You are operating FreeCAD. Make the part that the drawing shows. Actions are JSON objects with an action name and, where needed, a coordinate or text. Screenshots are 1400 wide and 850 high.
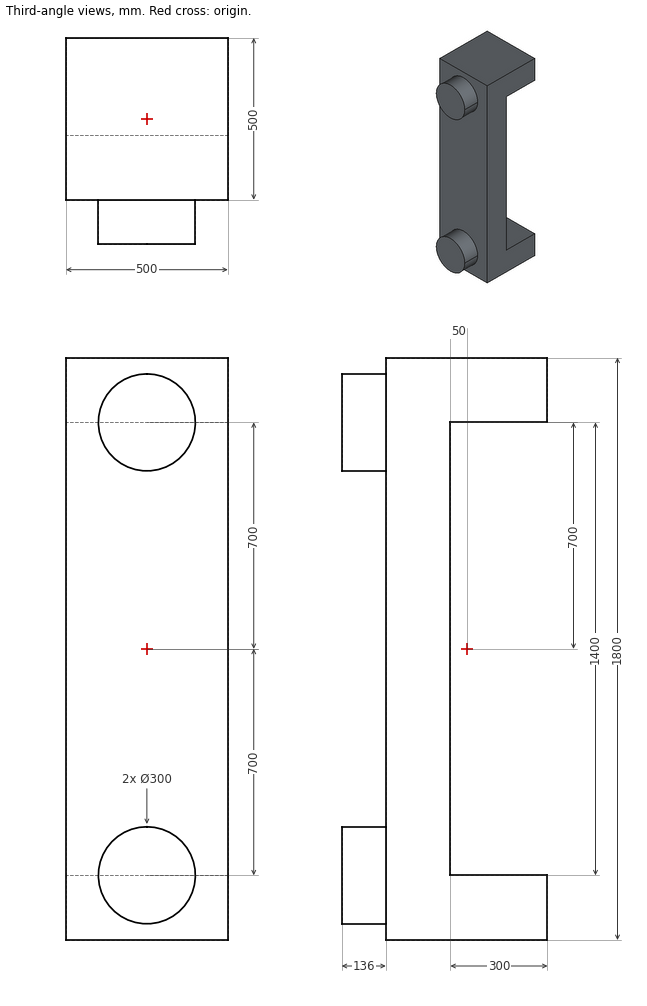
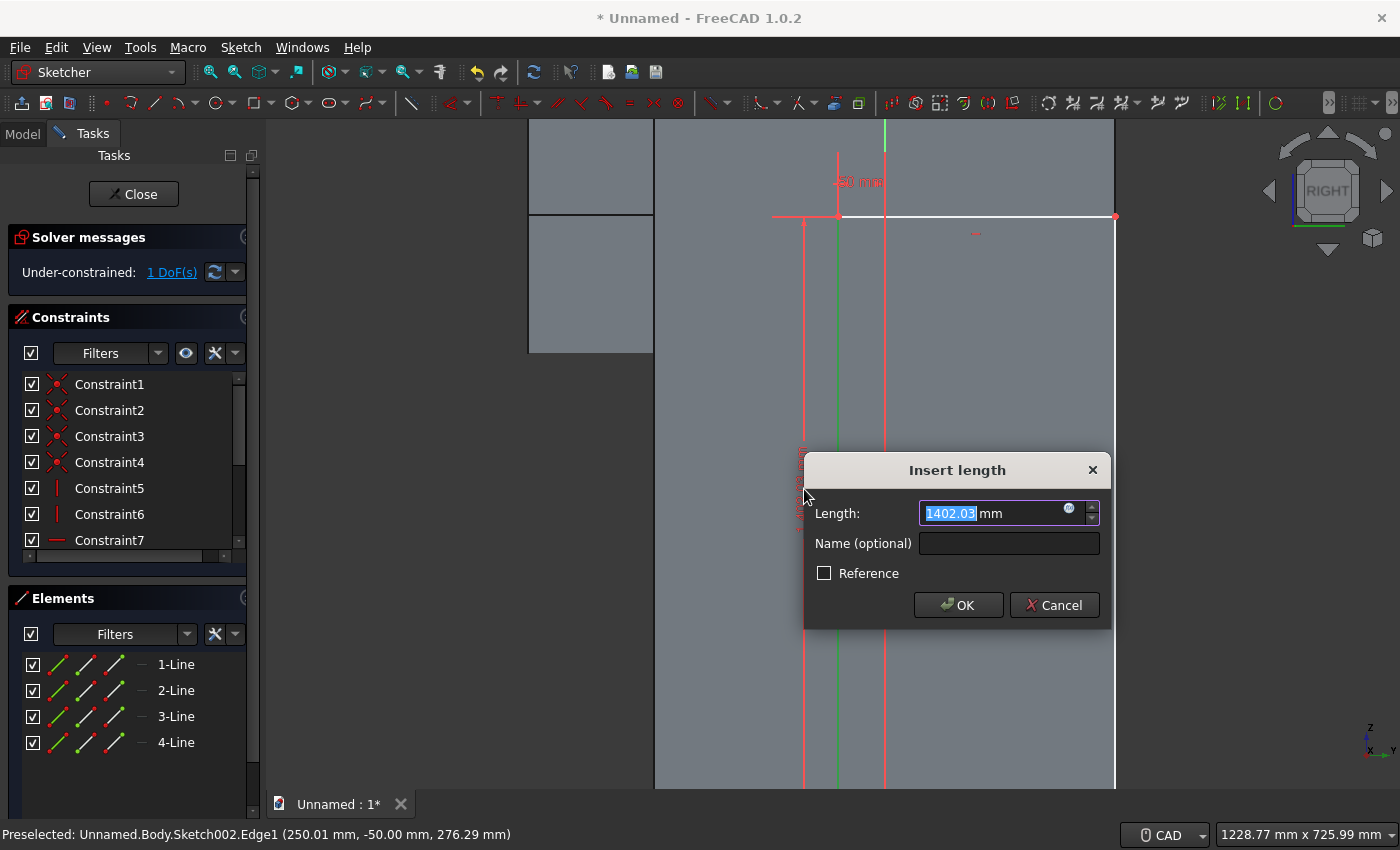
{"action": "type", "text": "1400"}
{"action": "key", "text": "Return"}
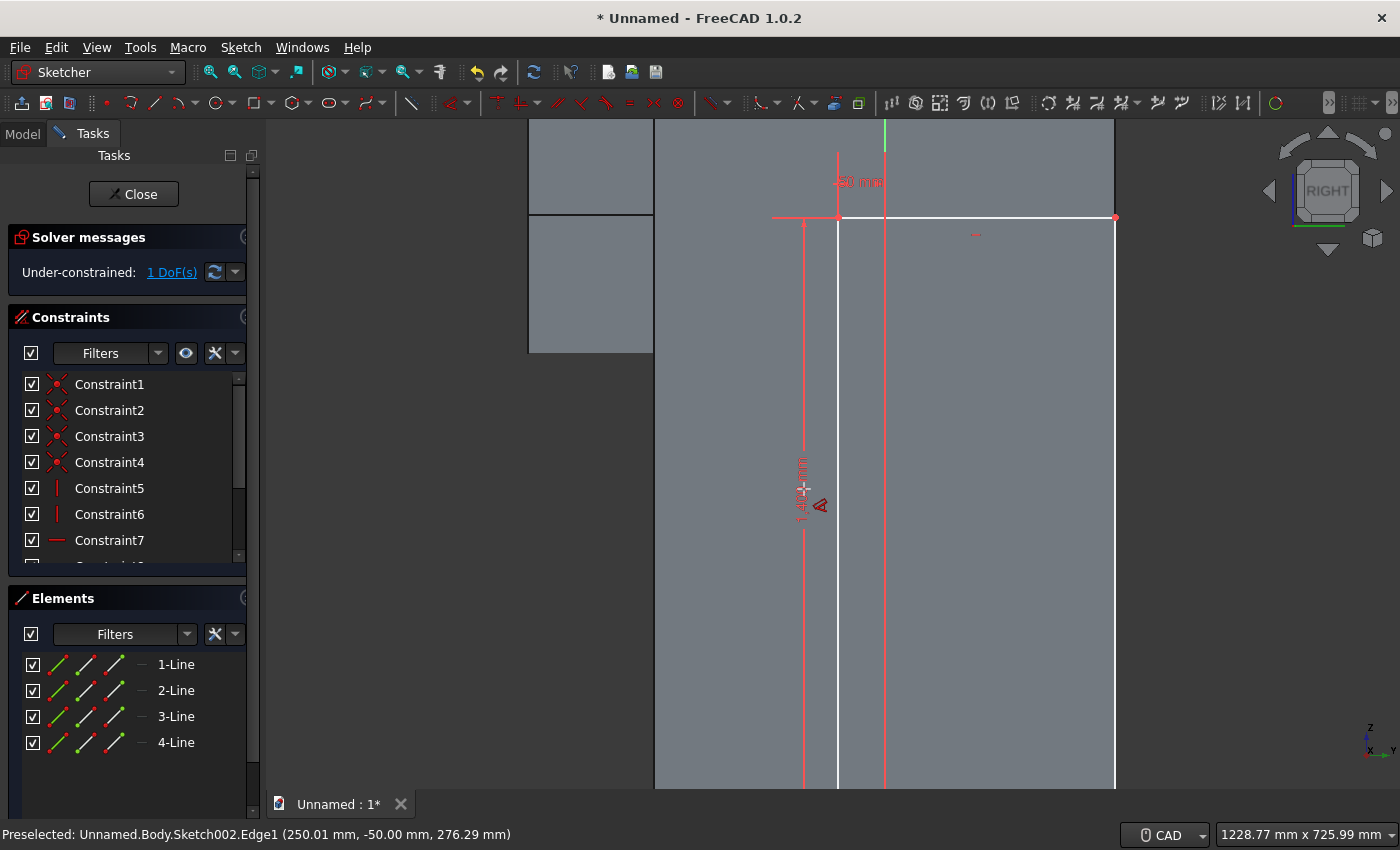
{"action": "left_click", "coordinate": [838, 218]}
{"action": "left_click", "coordinate": [804, 364]}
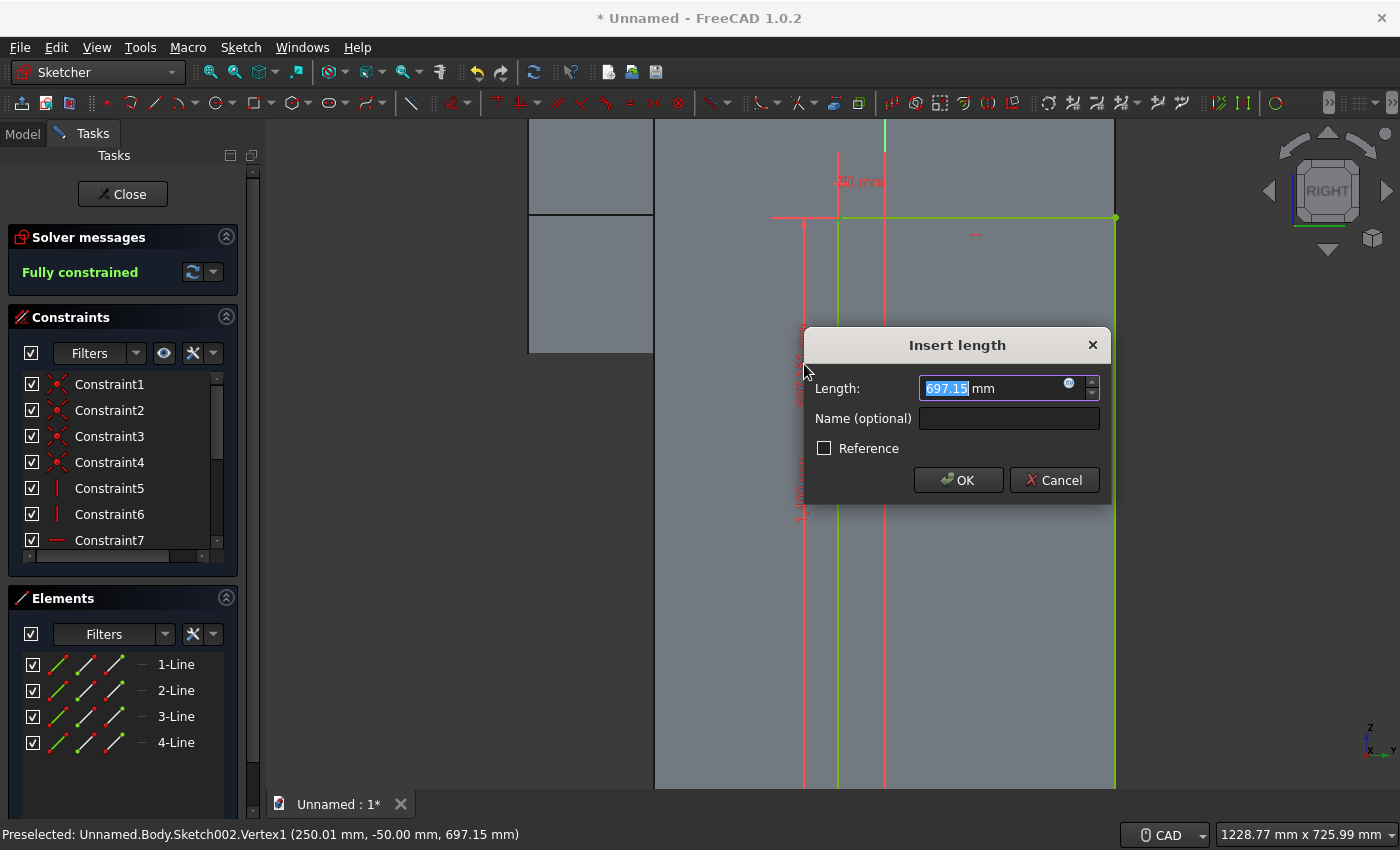
{"action": "type", "text": "700"}
{"action": "key", "text": "Return"}
{"action": "key", "text": "Escape"}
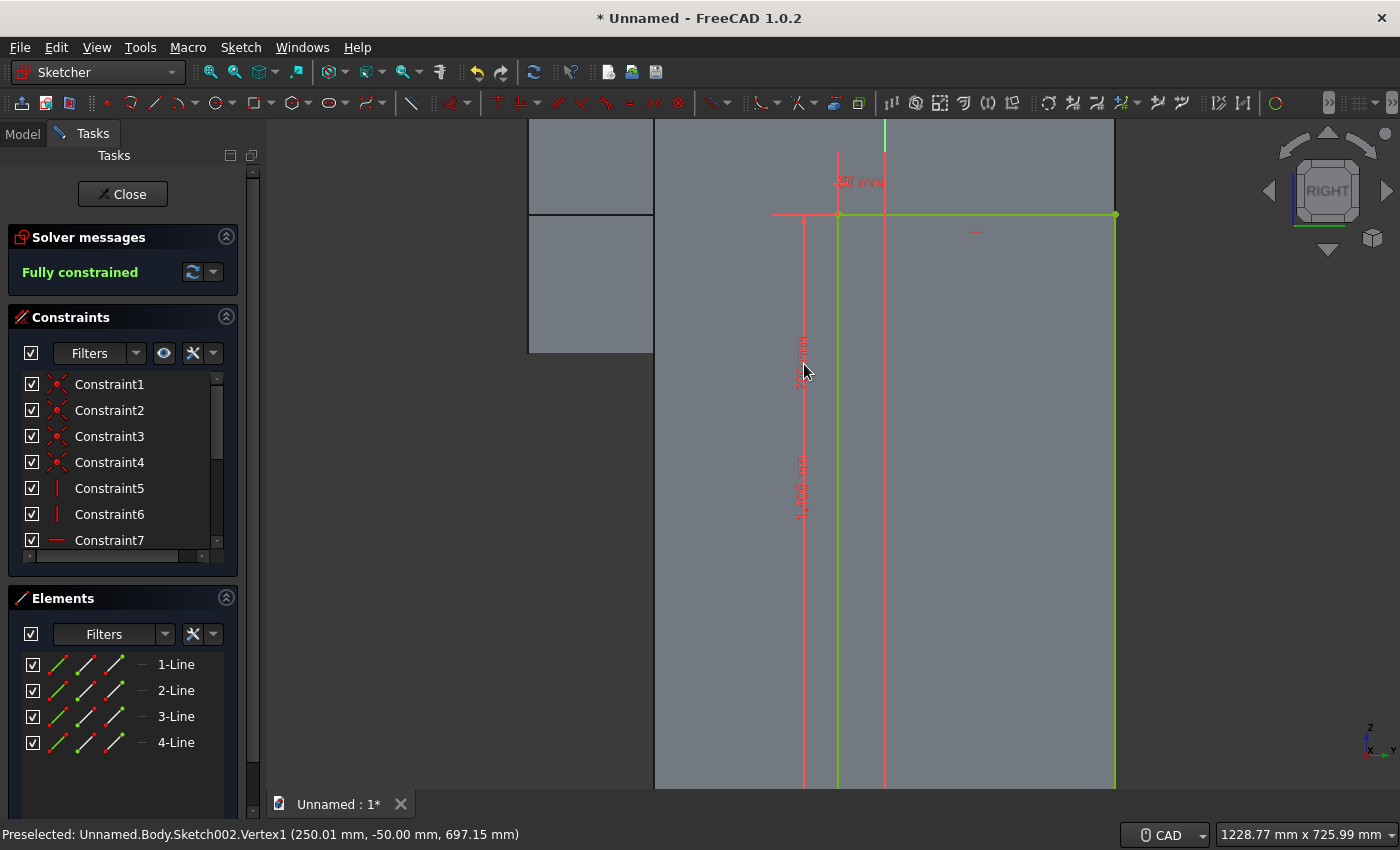
{"action": "left_click", "coordinate": [123, 194]}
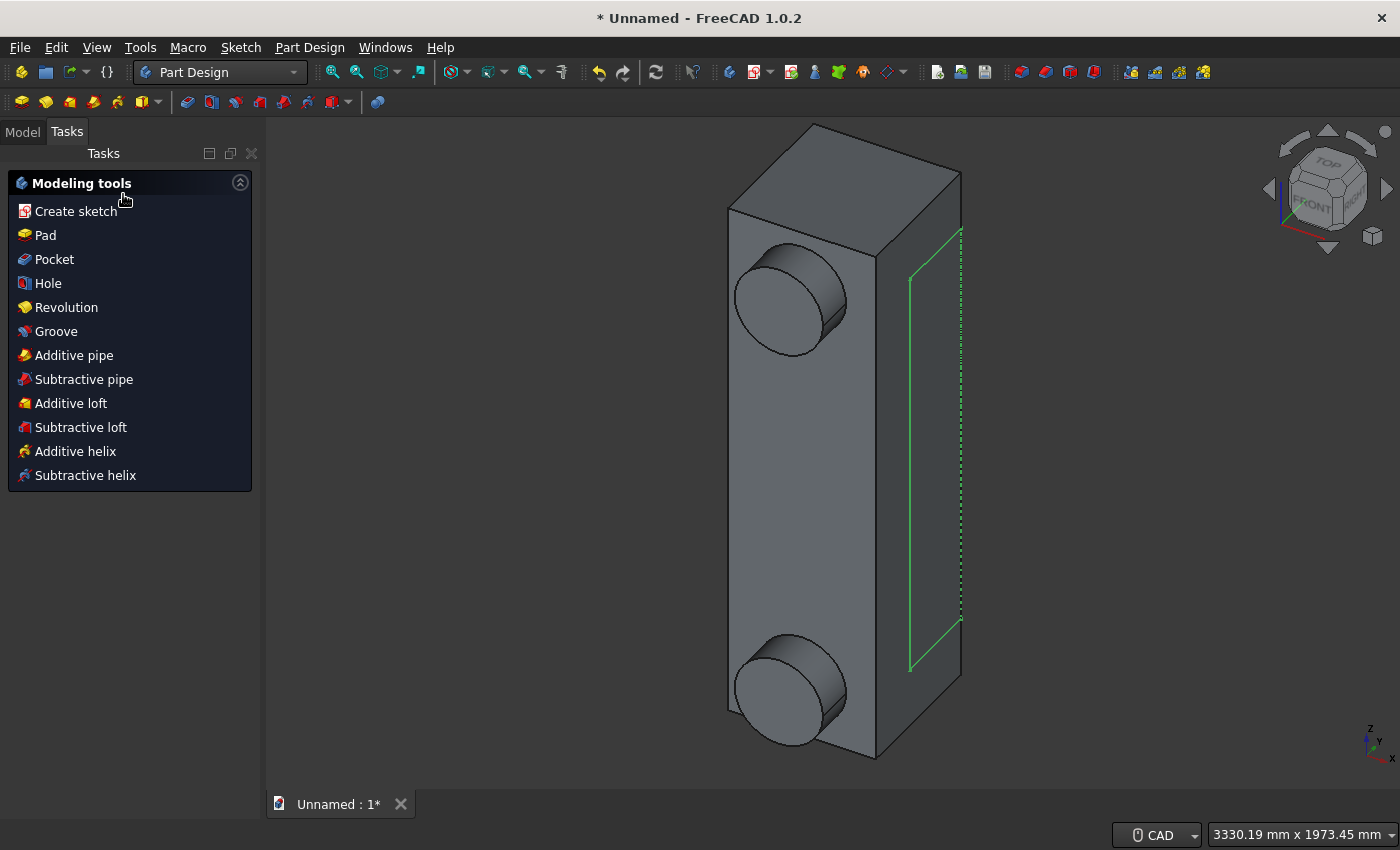
{"action": "left_click", "coordinate": [188, 102]}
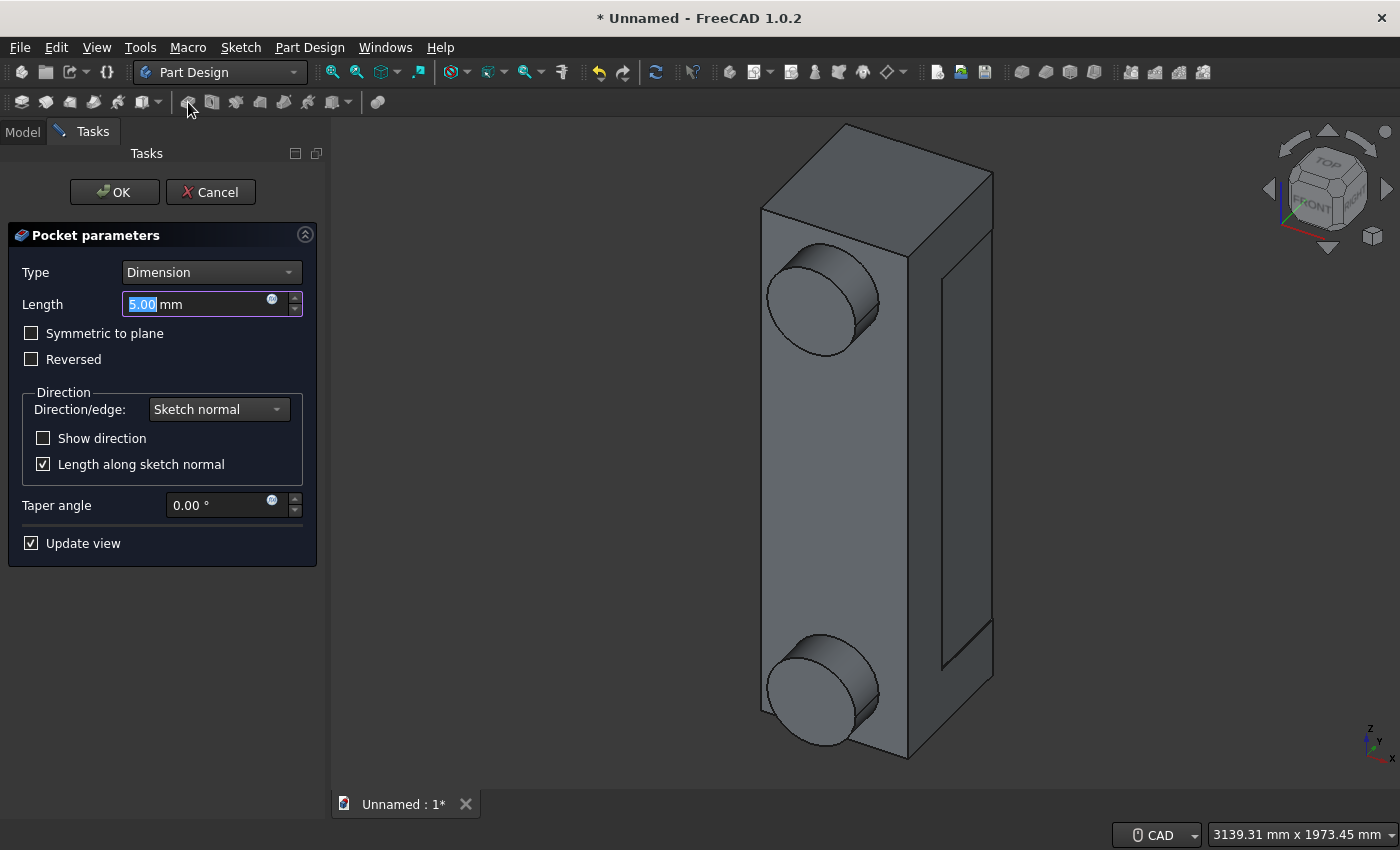
{"action": "left_click", "coordinate": [212, 272]}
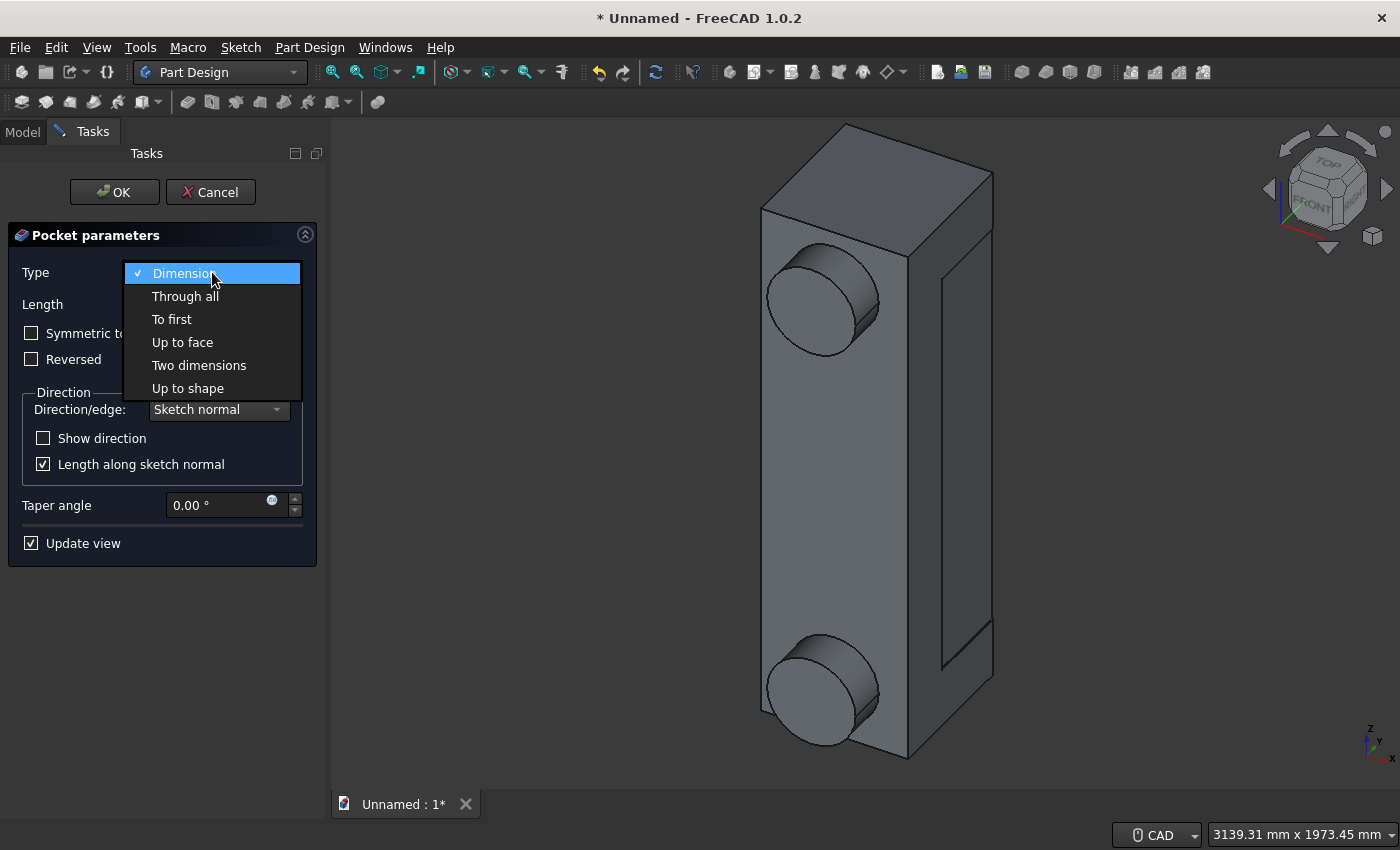
{"action": "left_click", "coordinate": [212, 296]}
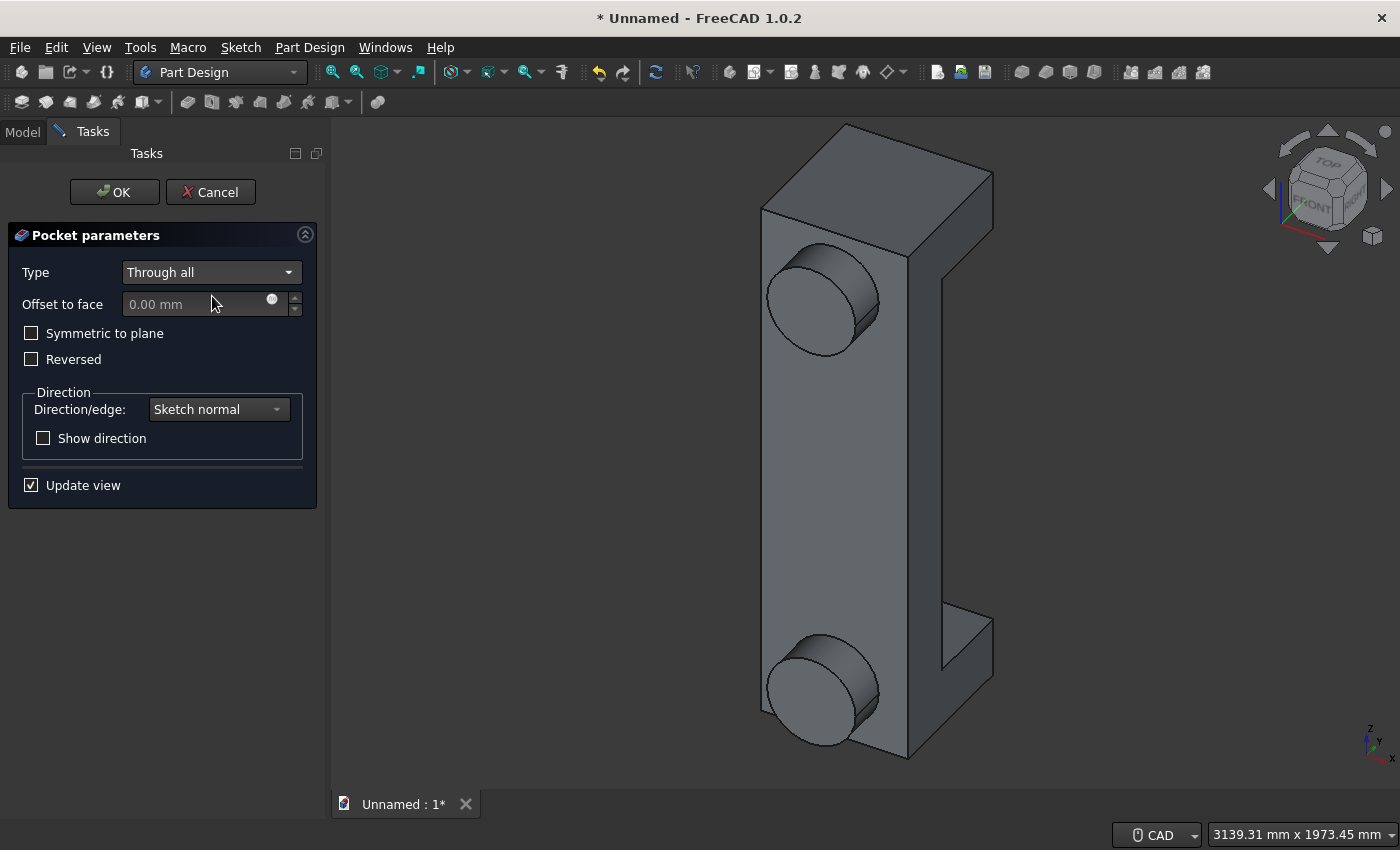
{"action": "left_click", "coordinate": [115, 192]}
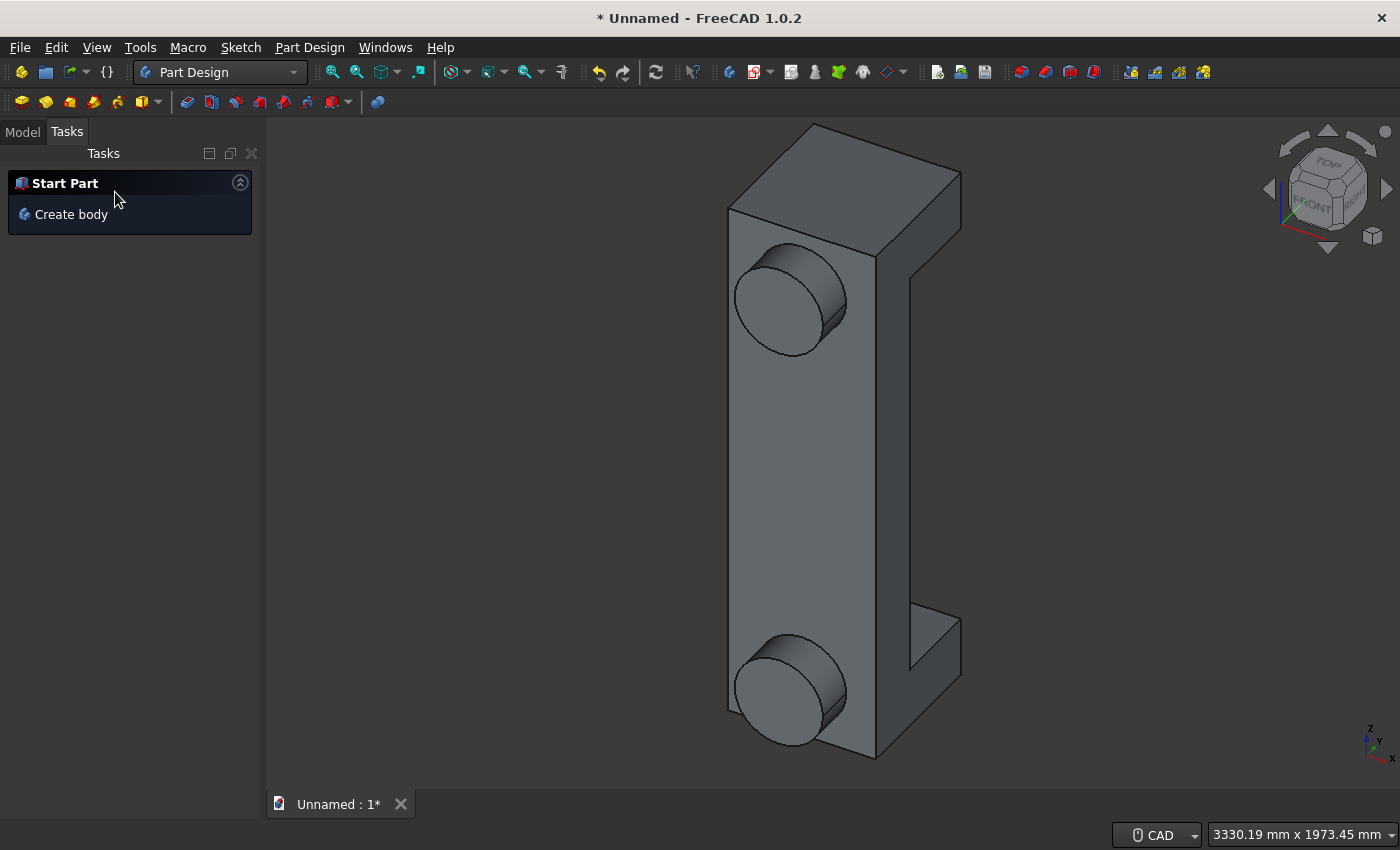
{"action": "key", "text": "0"}